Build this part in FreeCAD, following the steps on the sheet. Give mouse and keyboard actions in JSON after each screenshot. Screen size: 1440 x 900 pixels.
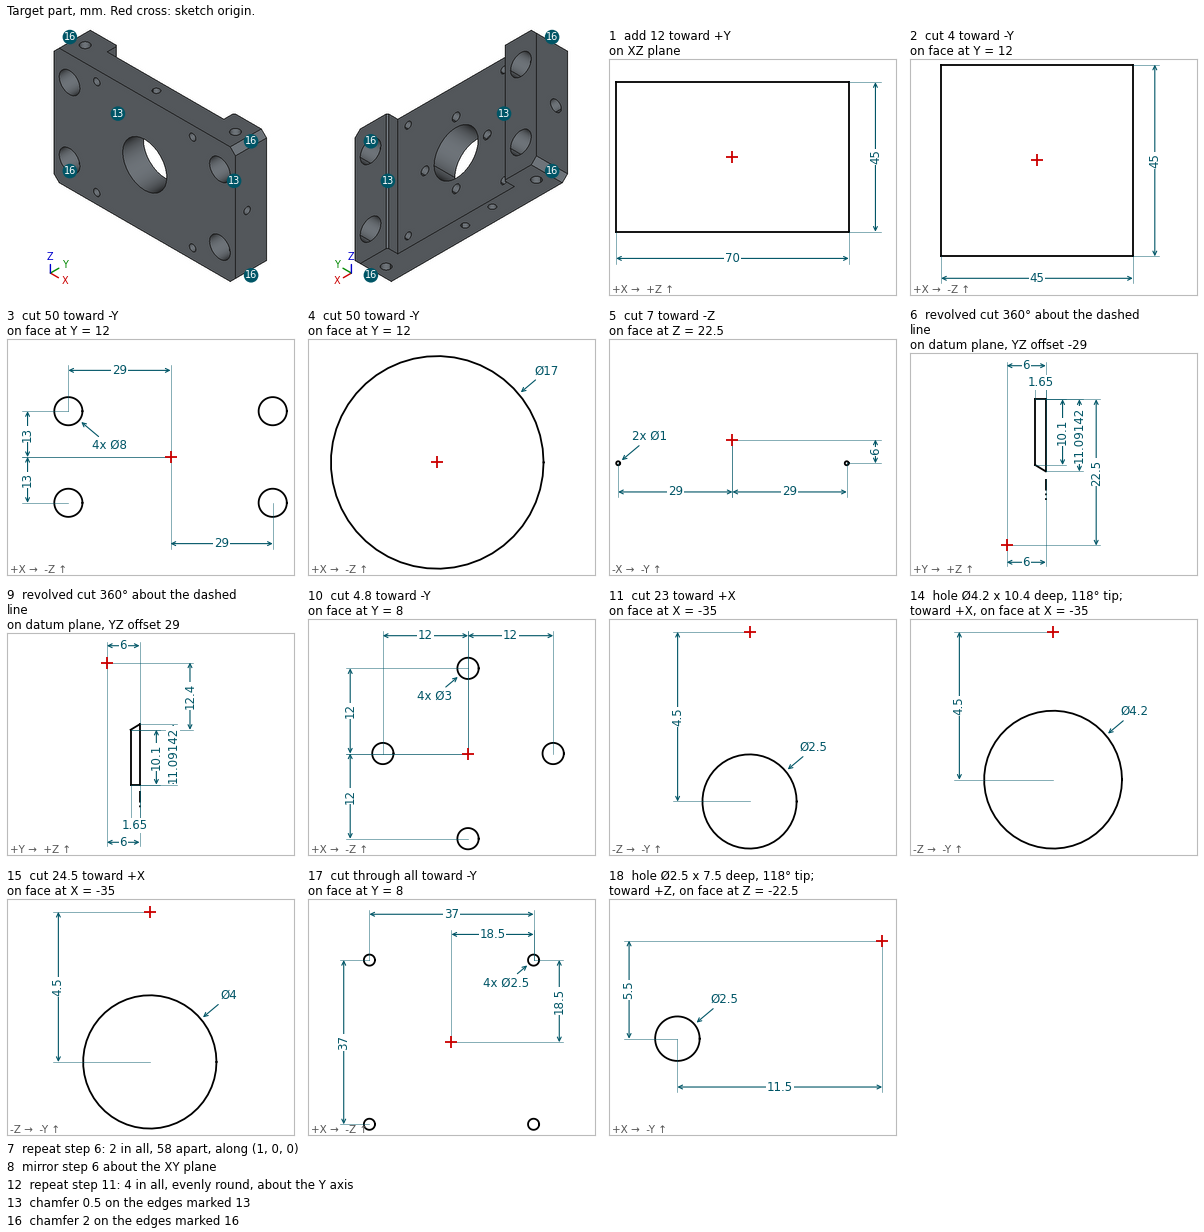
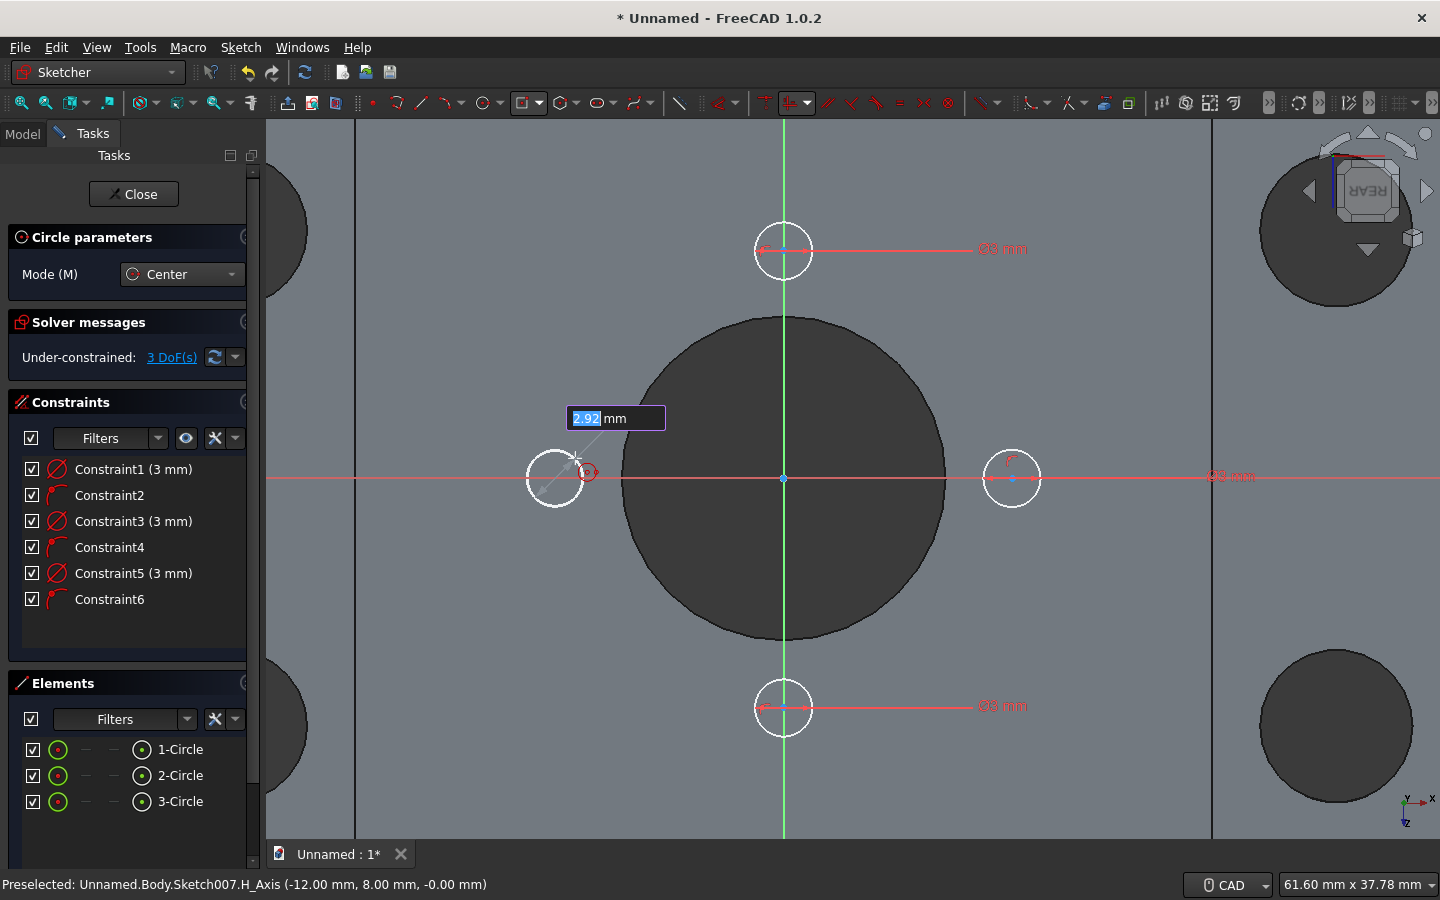
{"action": "type", "text": "3"}
{"action": "key", "text": "Return"}
{"action": "key", "text": "Escape"}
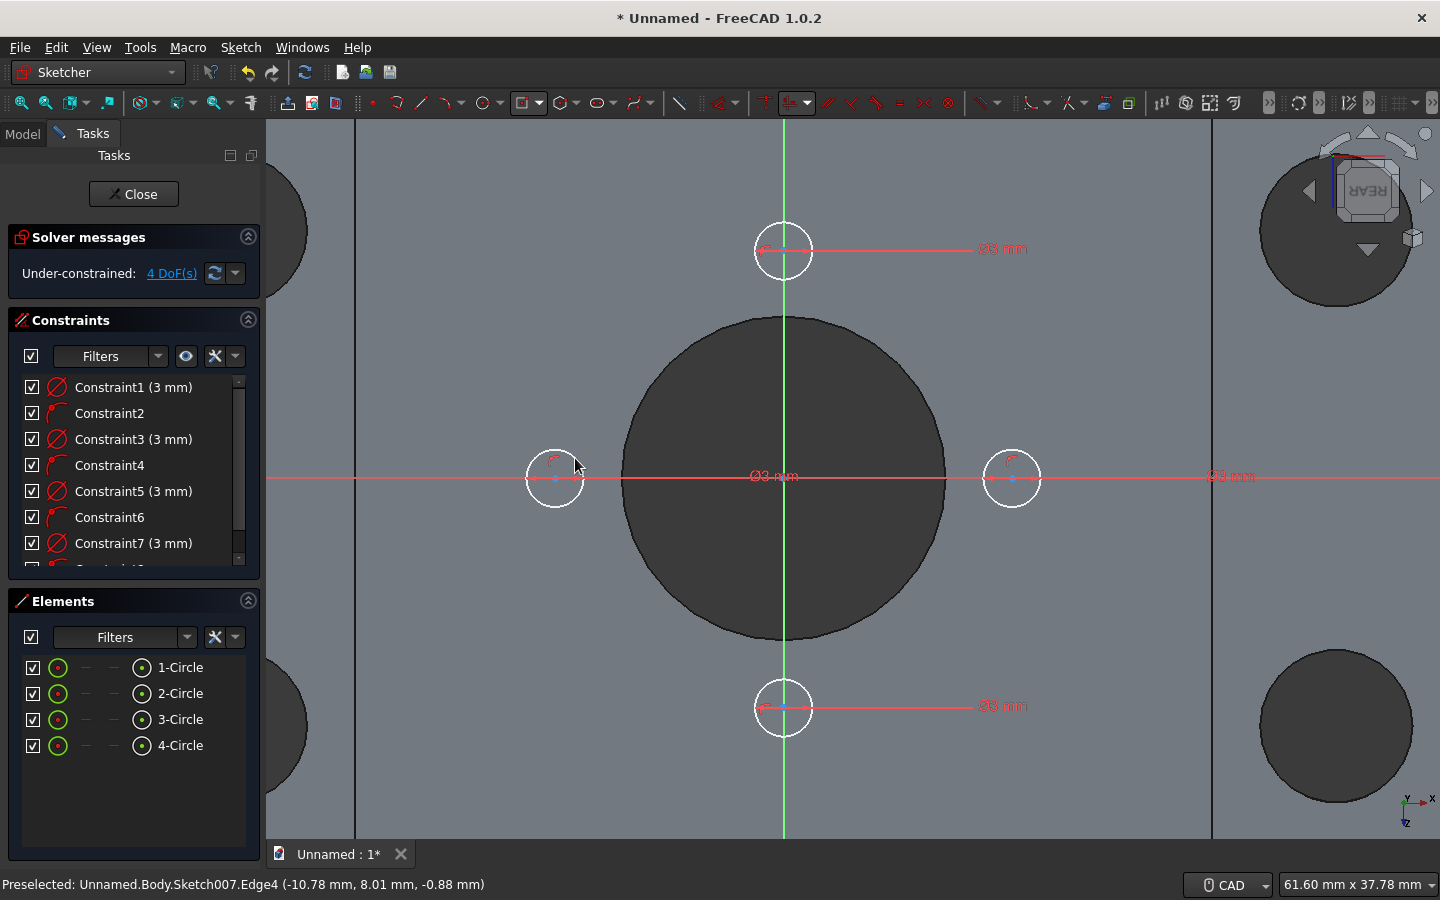
{"action": "left_click", "coordinate": [718, 104]}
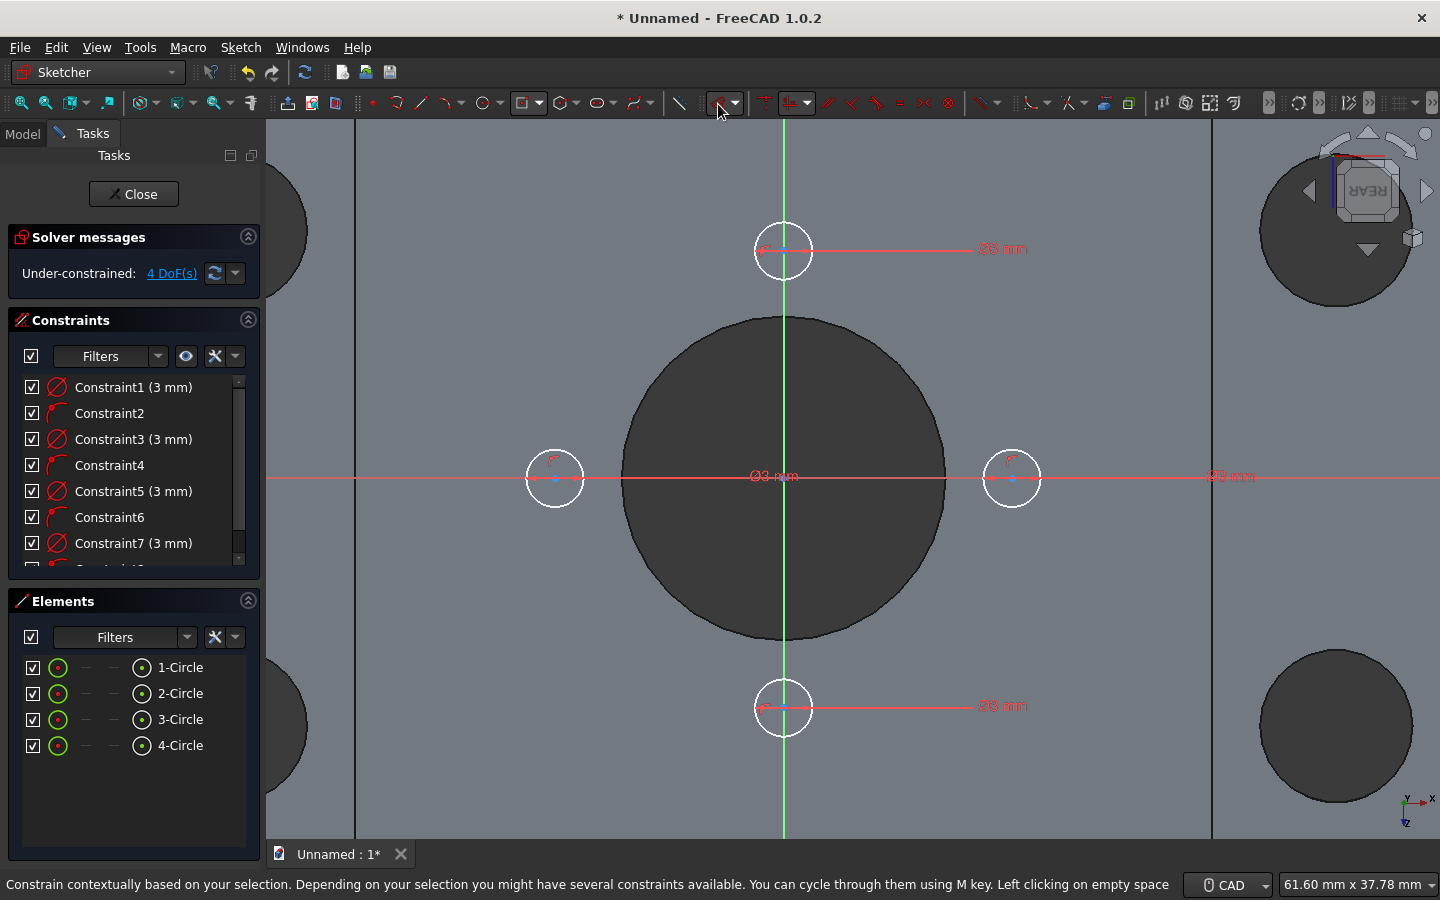
{"action": "left_click", "coordinate": [784, 251]}
{"action": "left_click", "coordinate": [818, 365]}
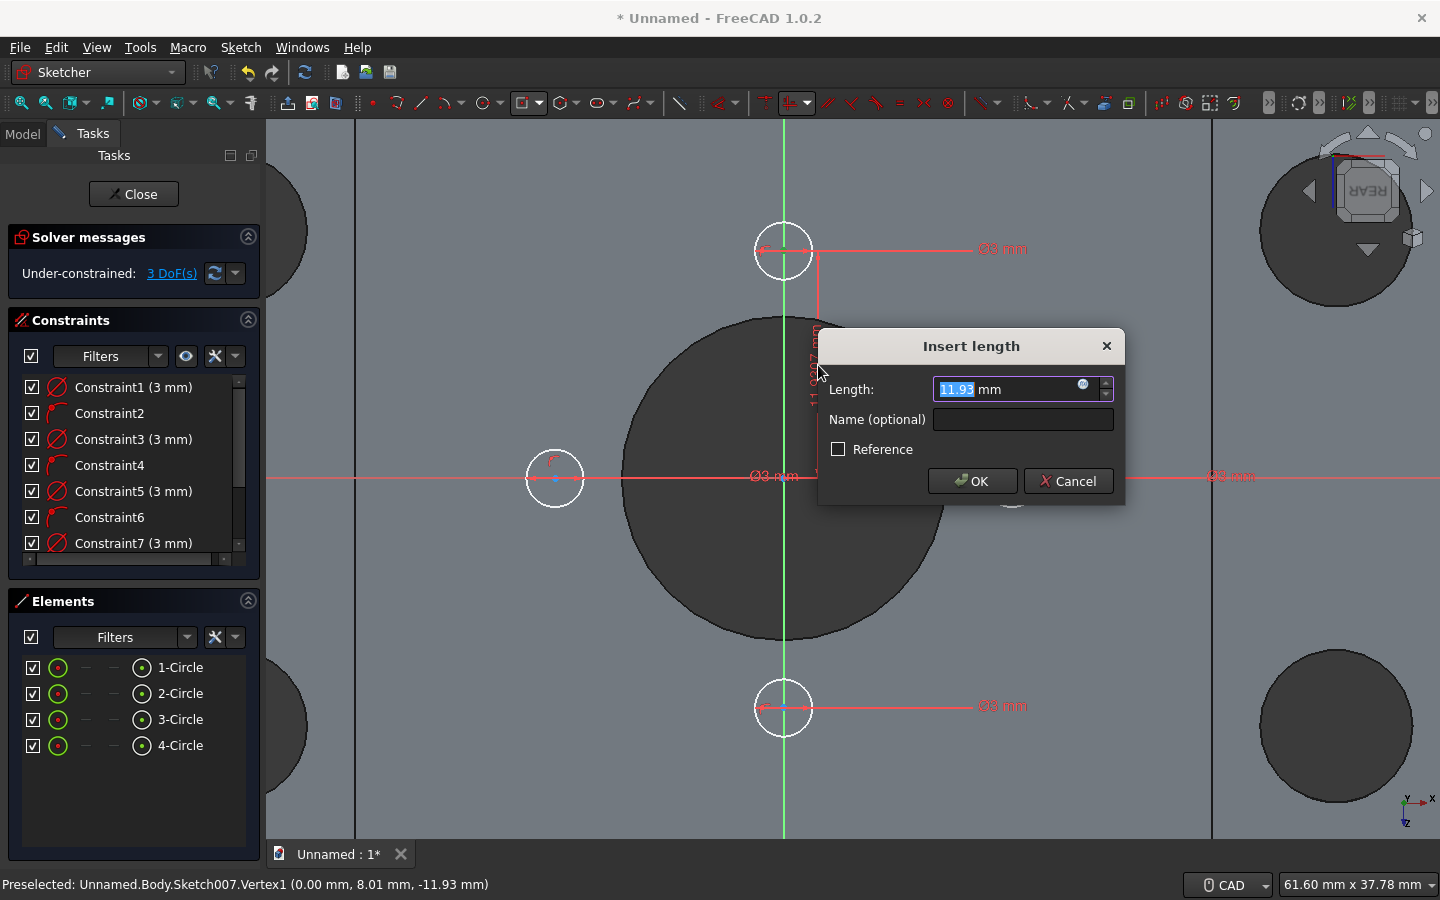
{"action": "type", "text": "12"}
{"action": "key", "text": "Return"}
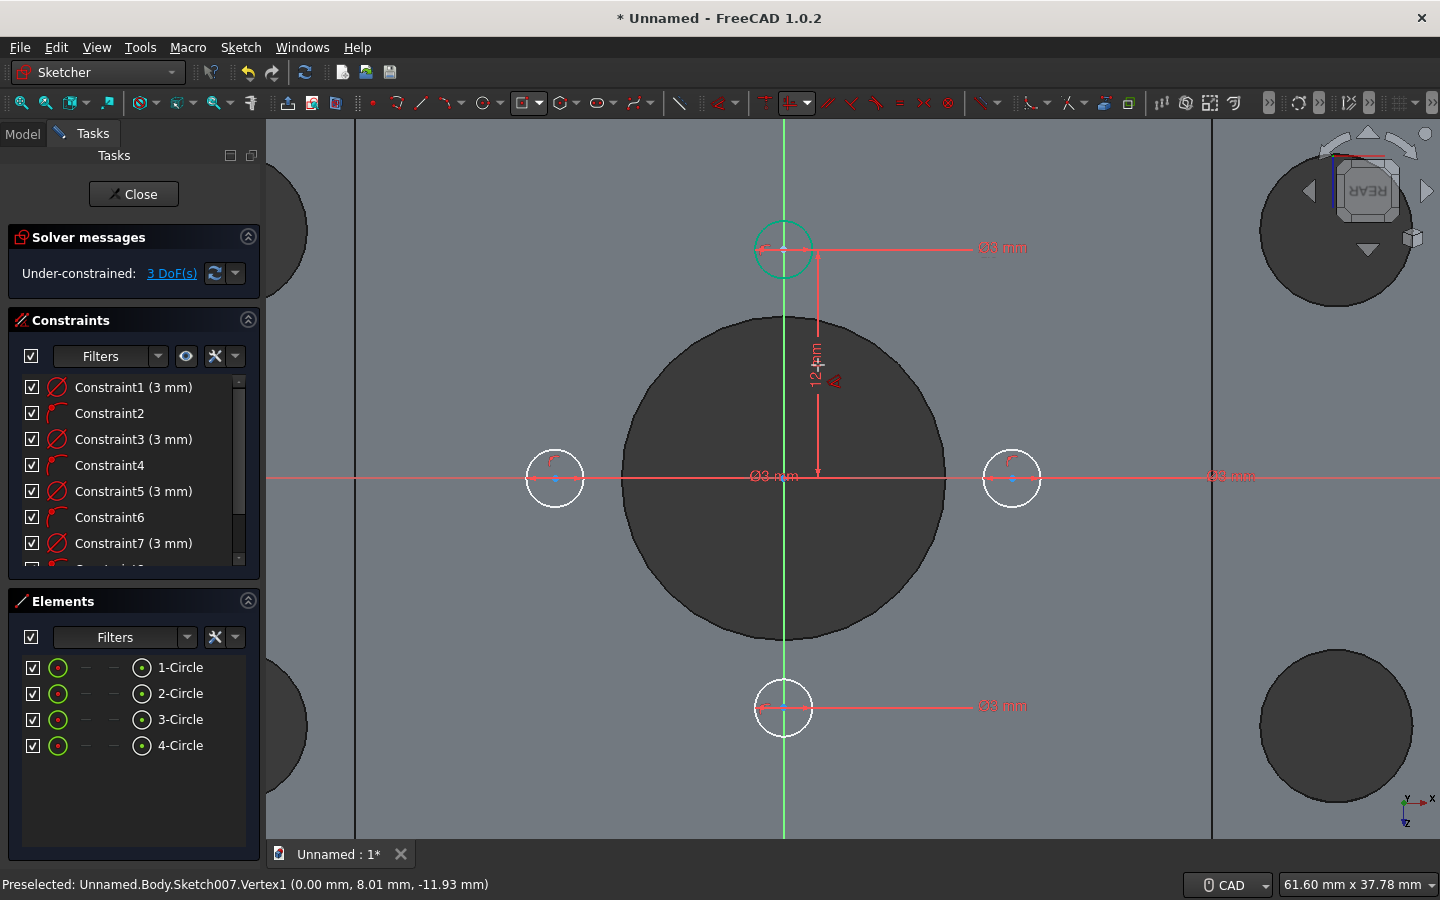
{"action": "left_click", "coordinate": [1012, 478]}
{"action": "left_click", "coordinate": [898, 512]}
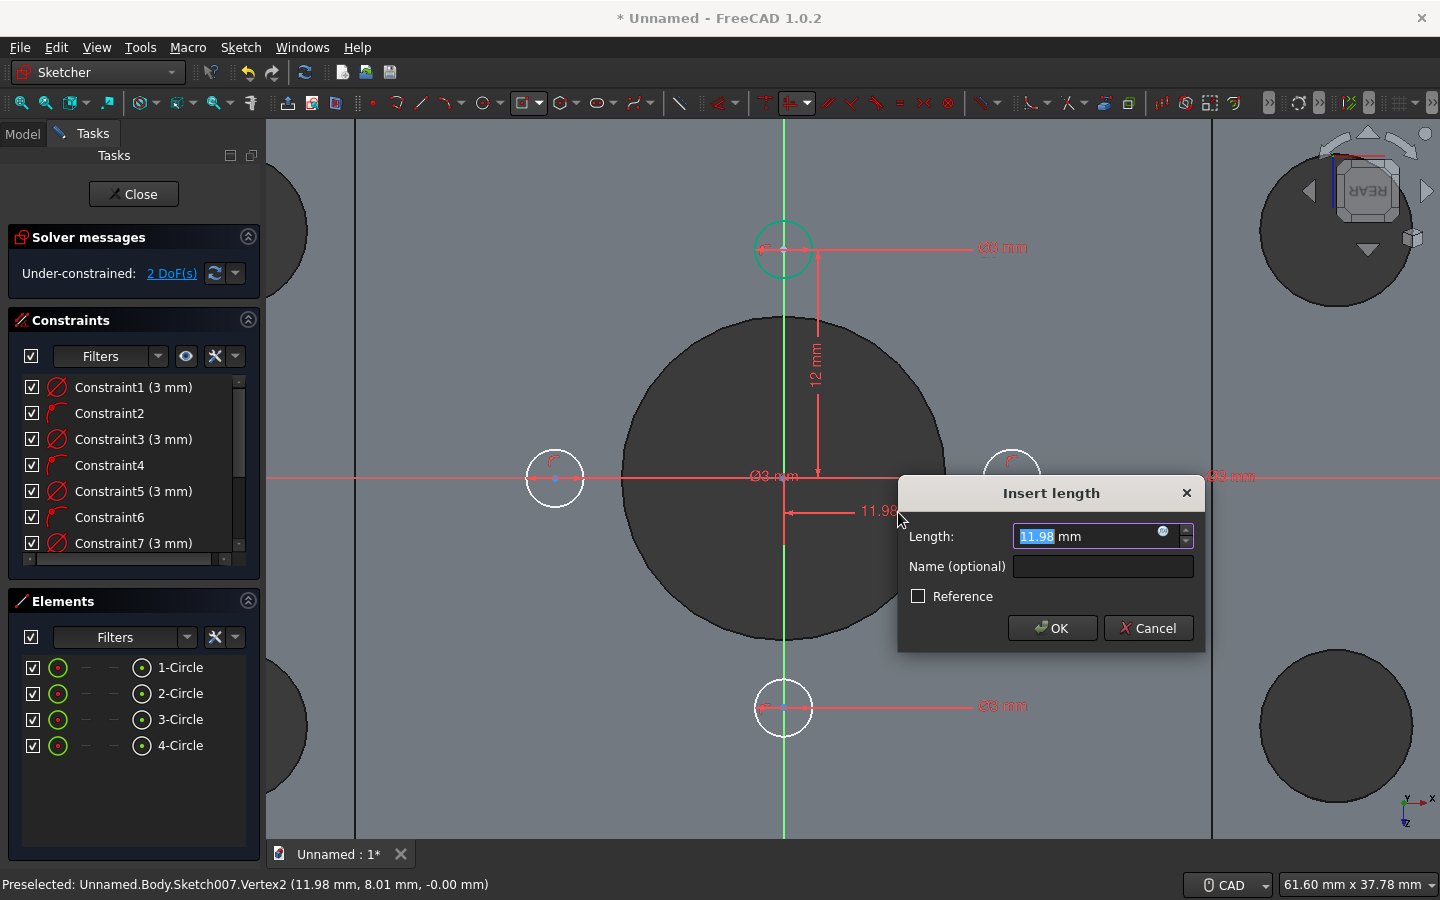
{"action": "type", "text": "12"}
{"action": "key", "text": "Return"}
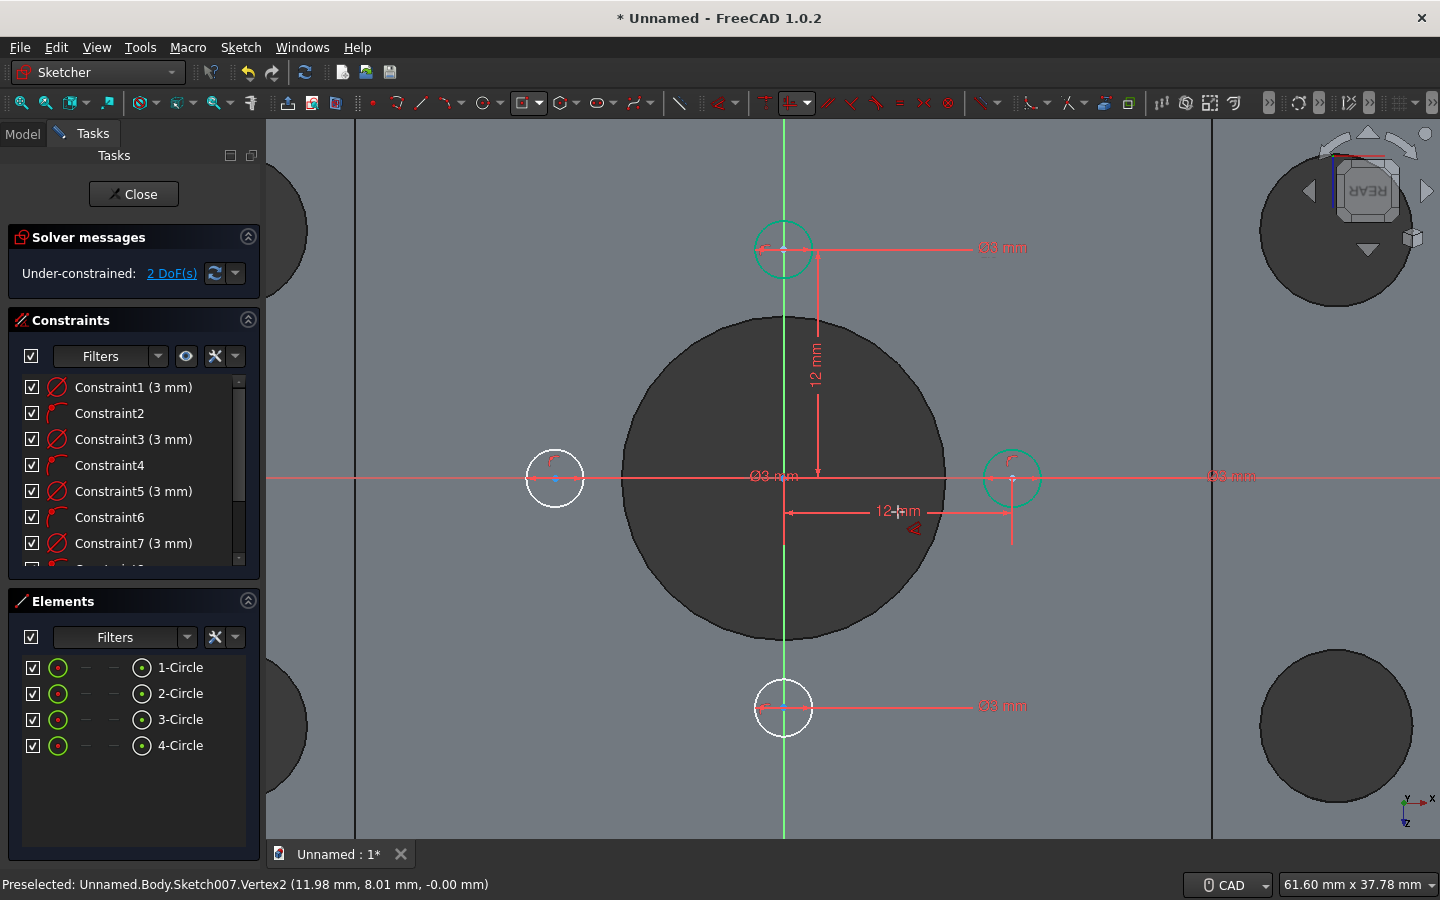
{"action": "left_click", "coordinate": [784, 708]}
{"action": "left_click", "coordinate": [818, 593]}